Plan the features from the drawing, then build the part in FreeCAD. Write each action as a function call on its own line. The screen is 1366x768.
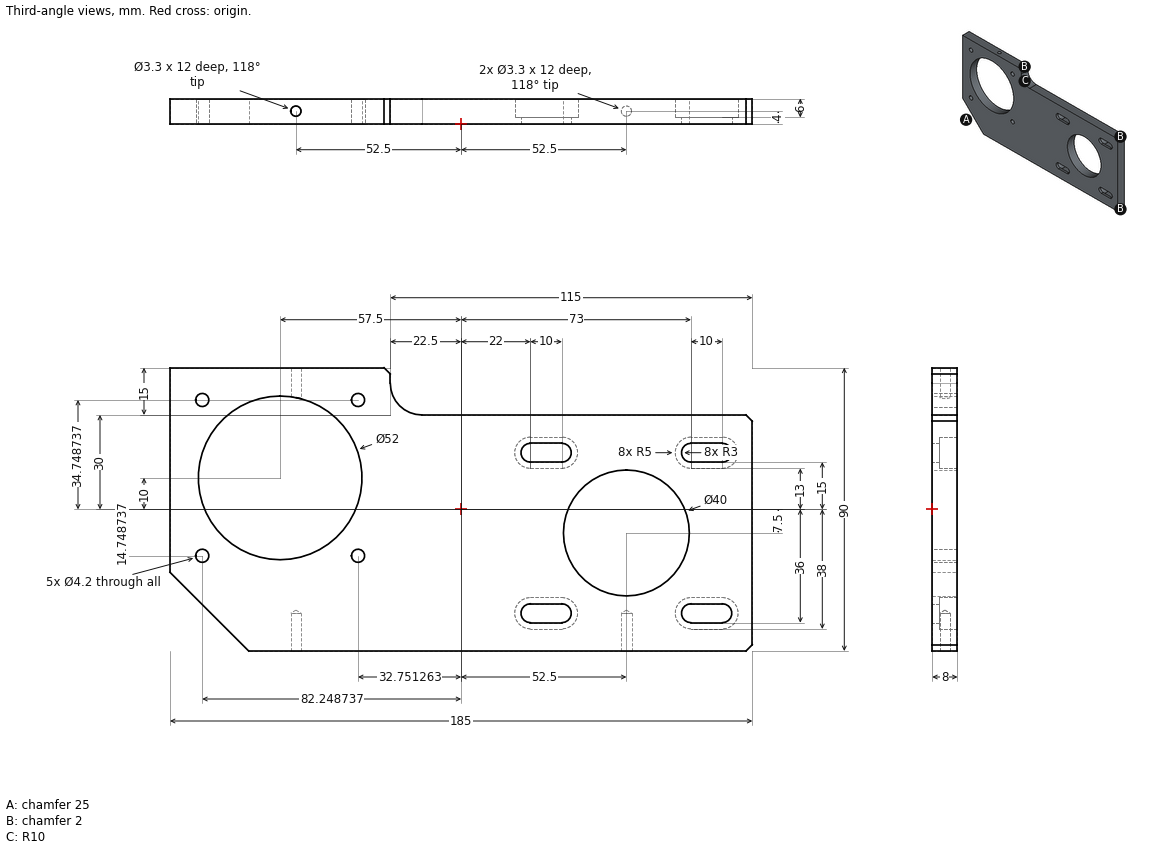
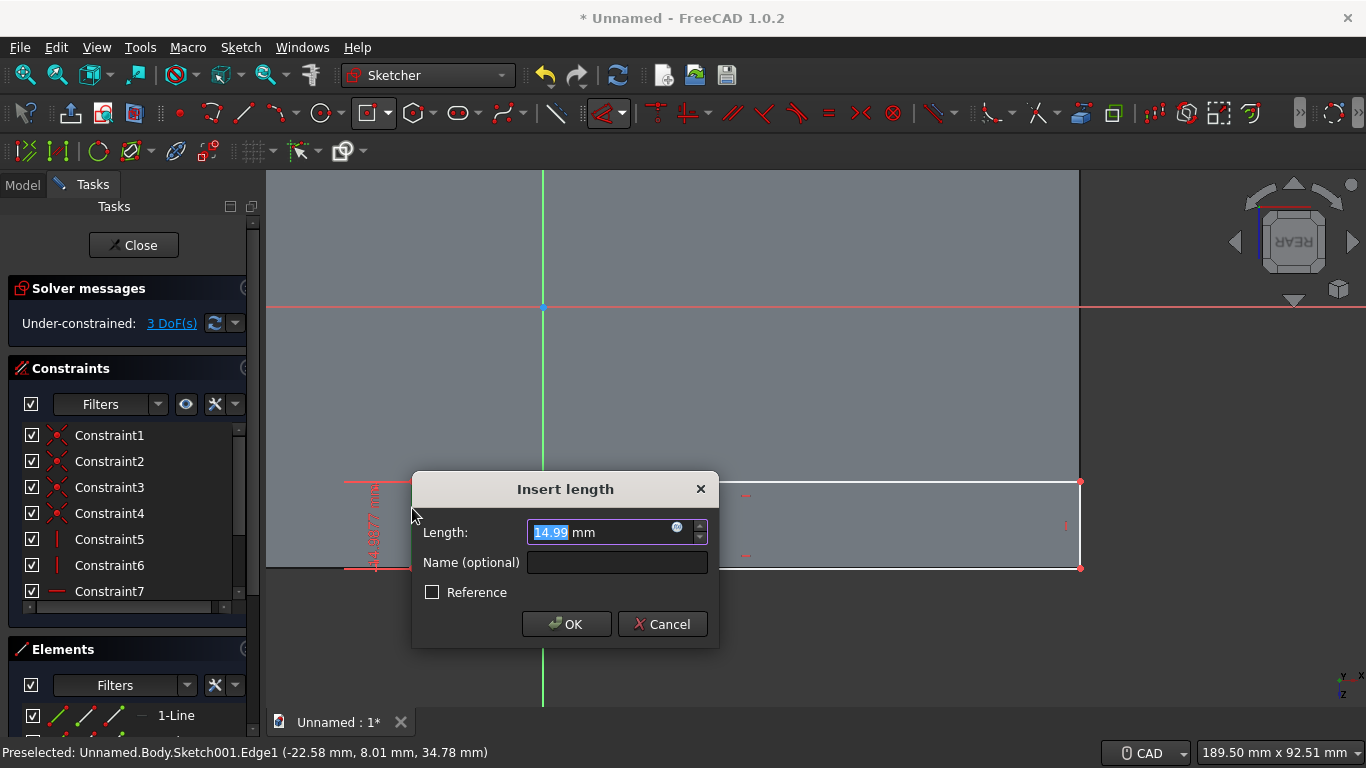
text(15)
key(Return)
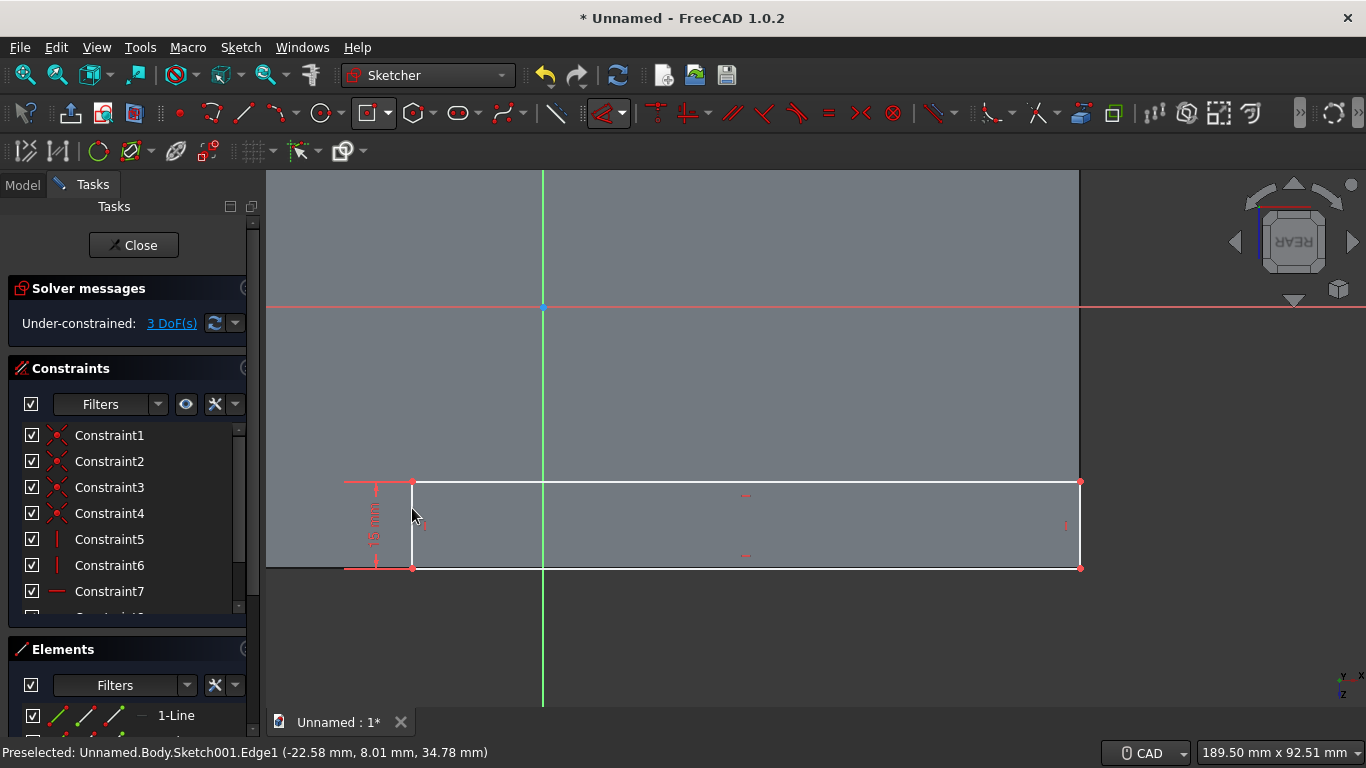
click(612, 569)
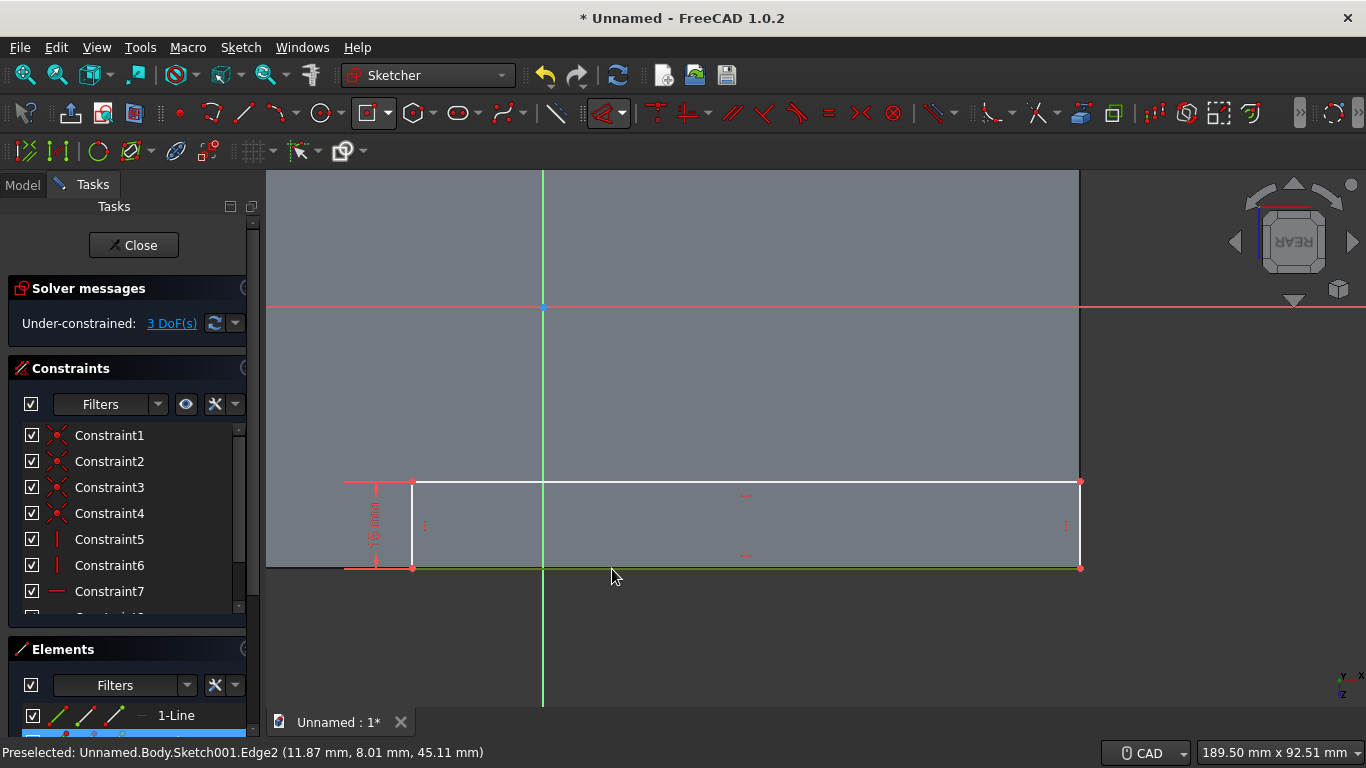
key(l)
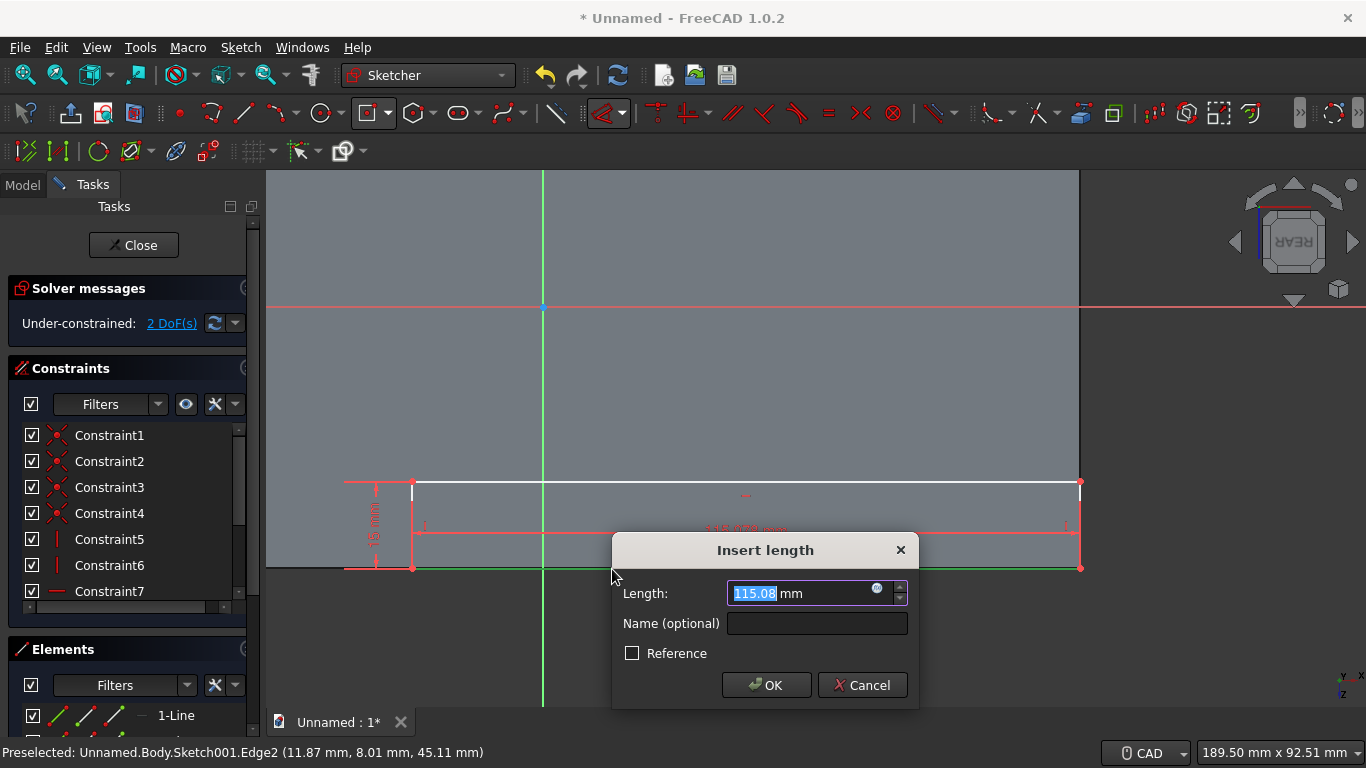
text(115)
key(Return)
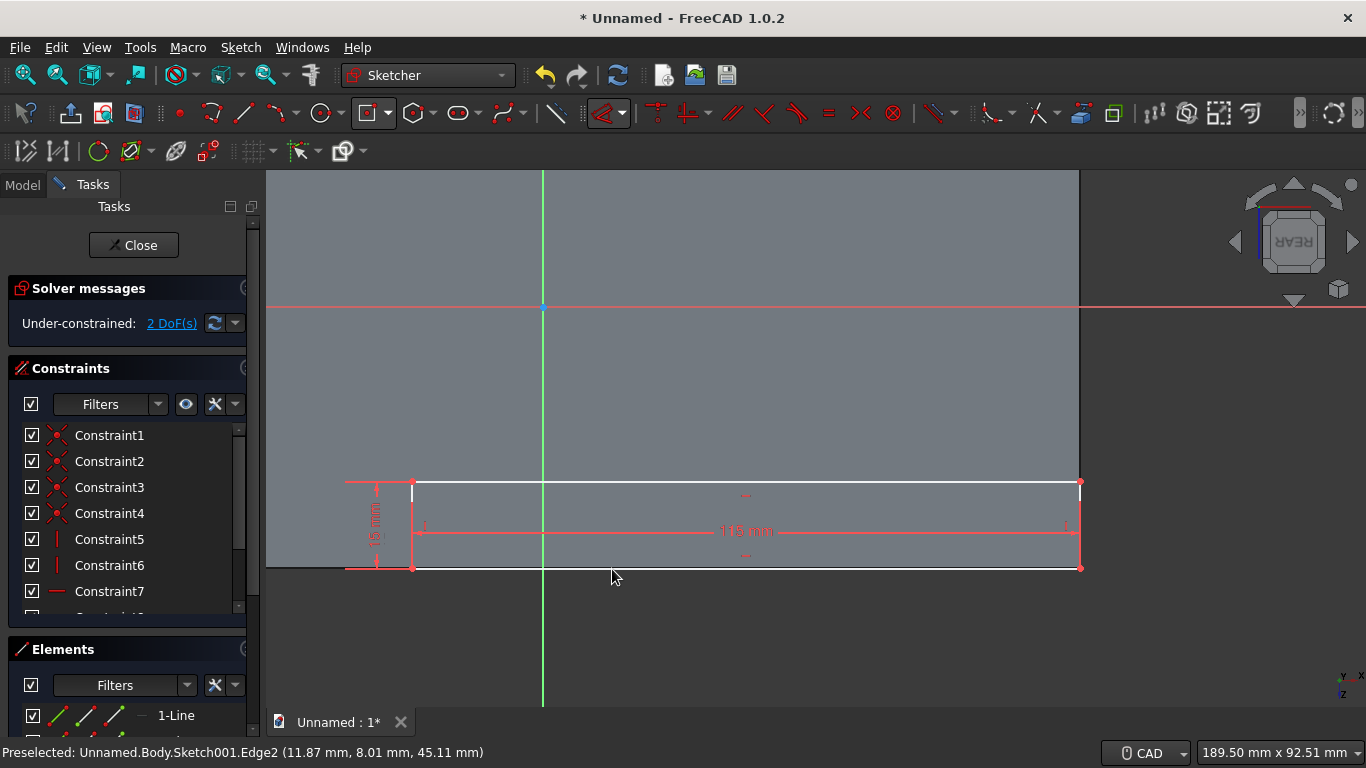
click(412, 482)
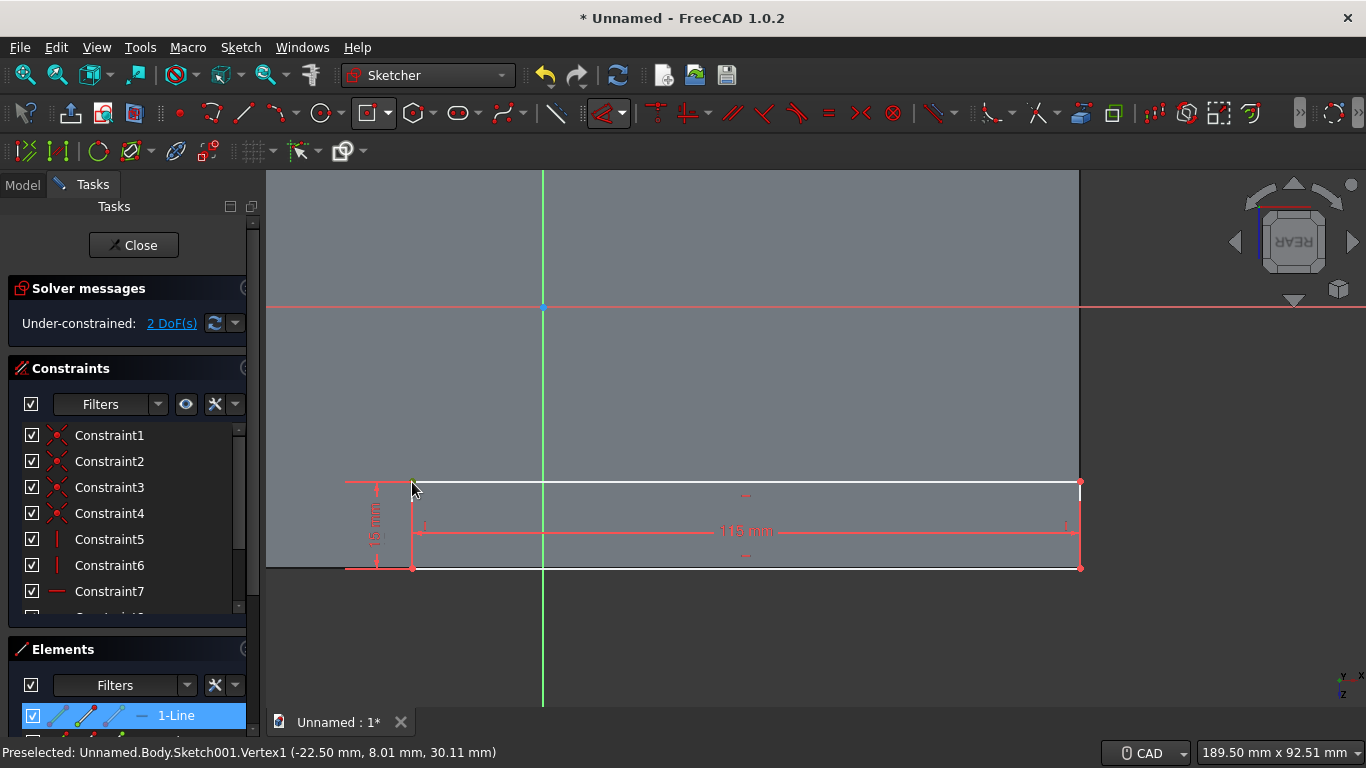
click(624, 114)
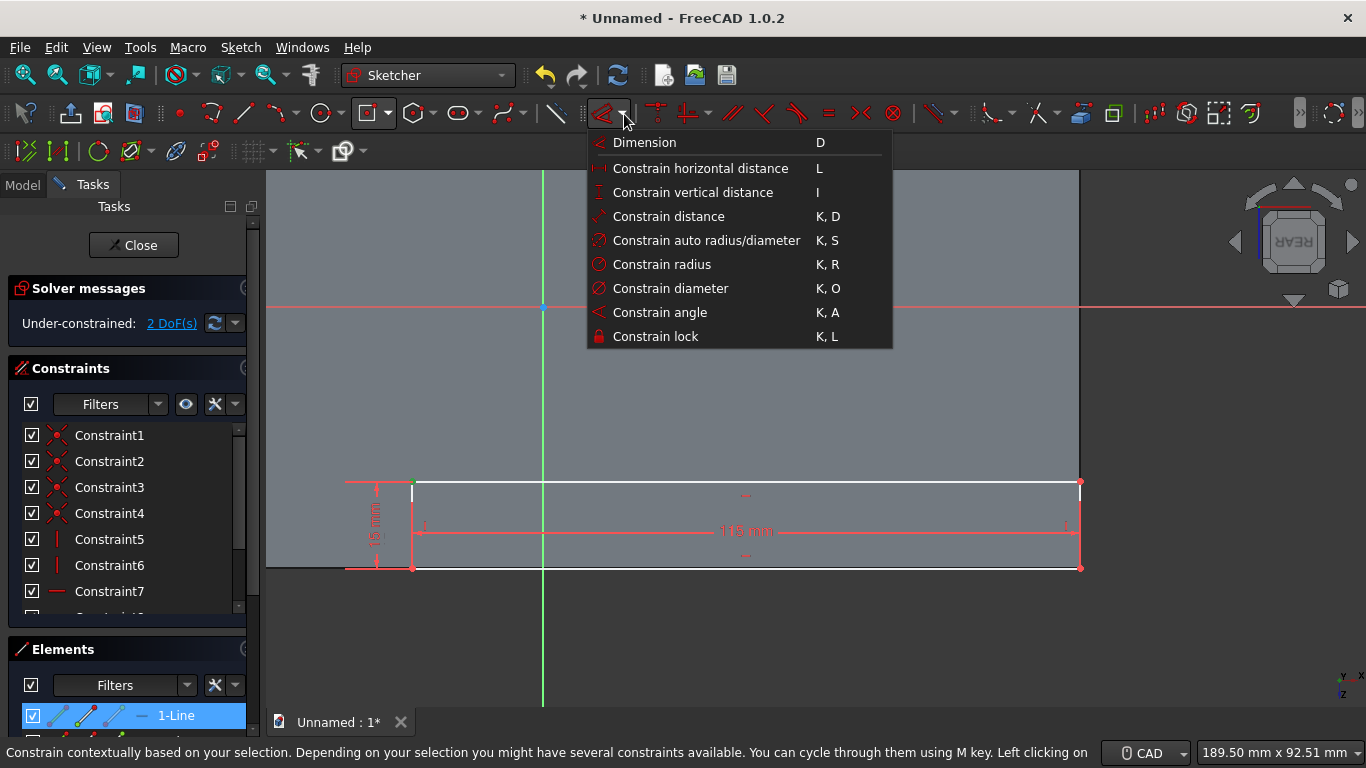
click(740, 192)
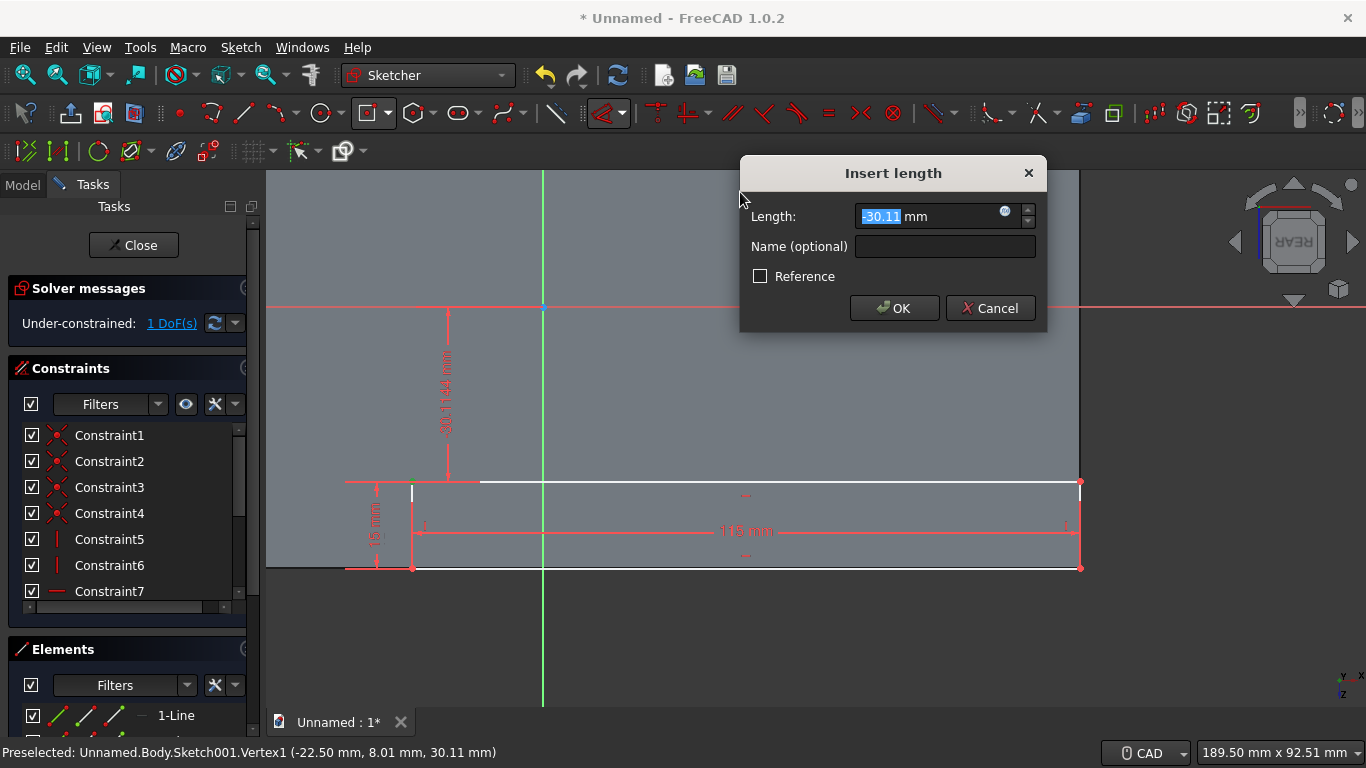
text(-30)
key(Return)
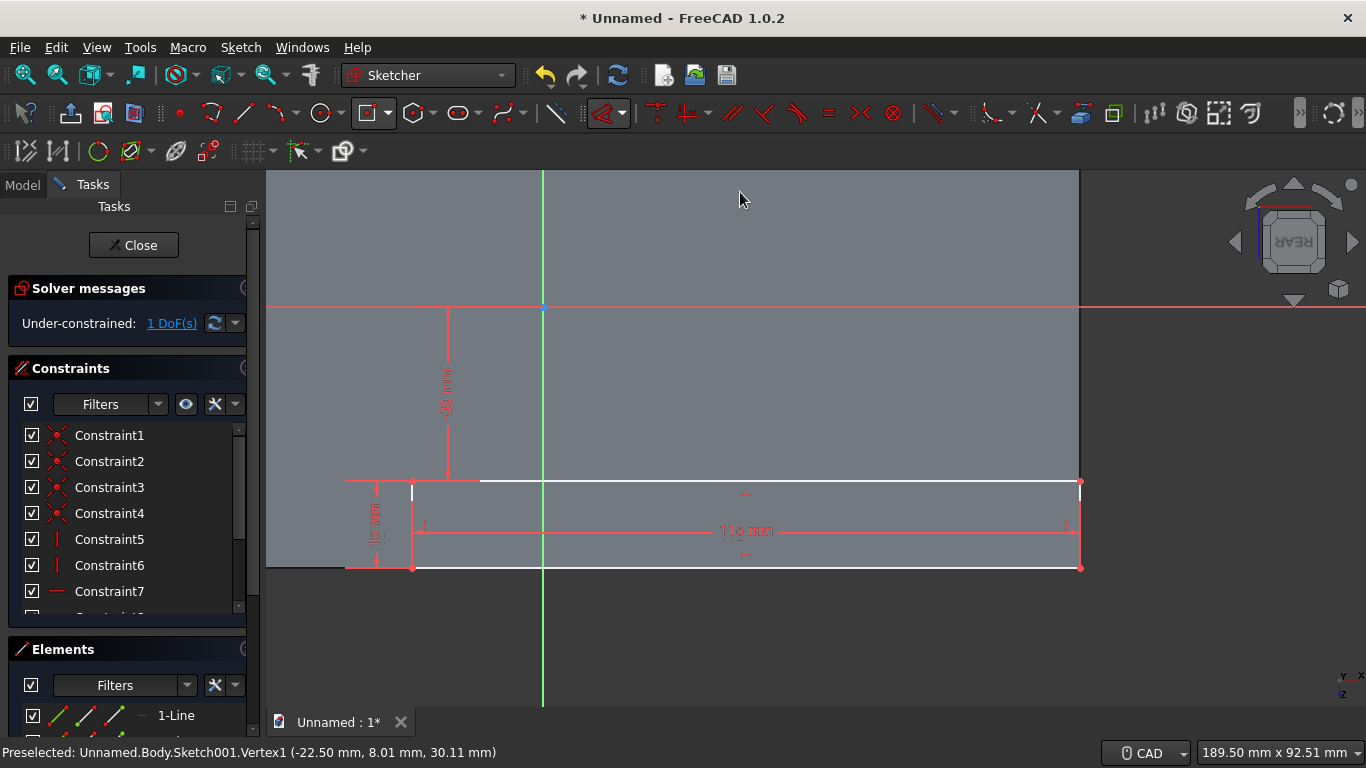
click(412, 481)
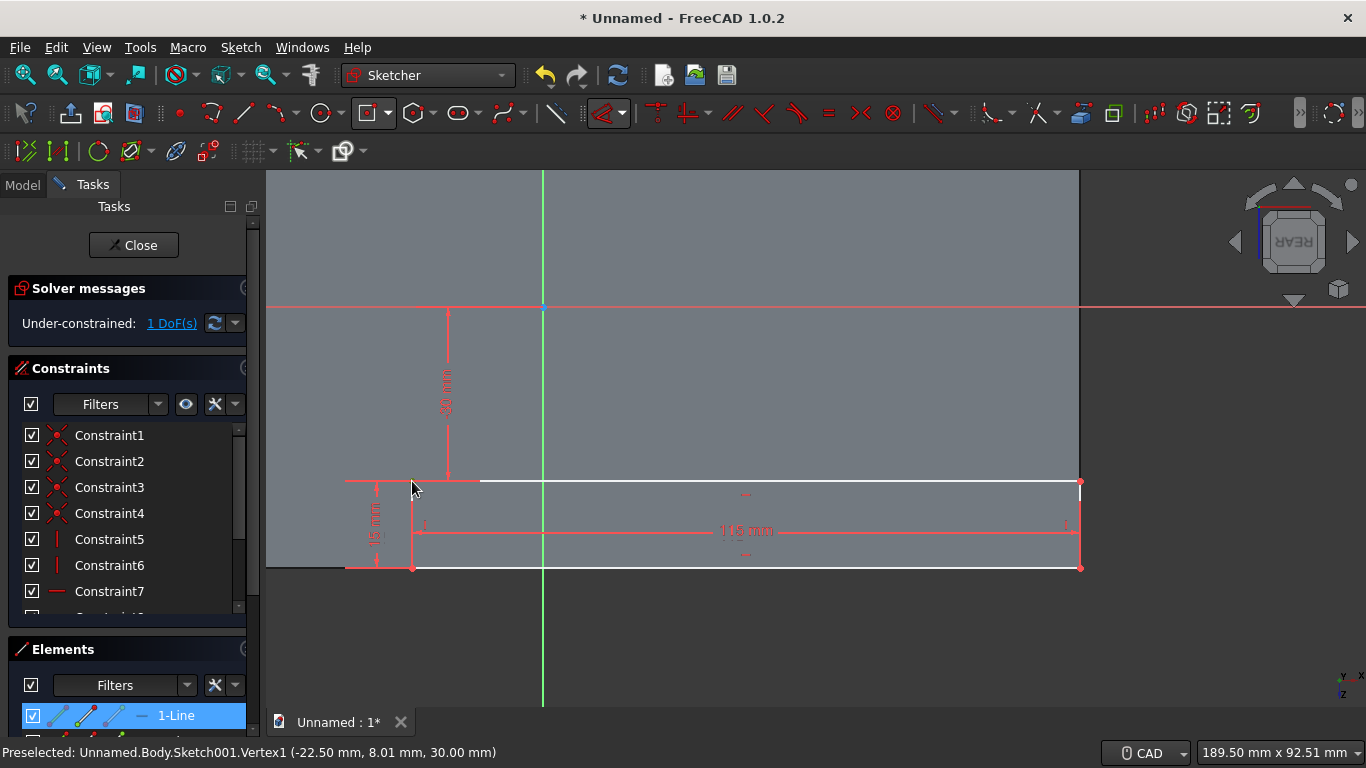
click(624, 114)